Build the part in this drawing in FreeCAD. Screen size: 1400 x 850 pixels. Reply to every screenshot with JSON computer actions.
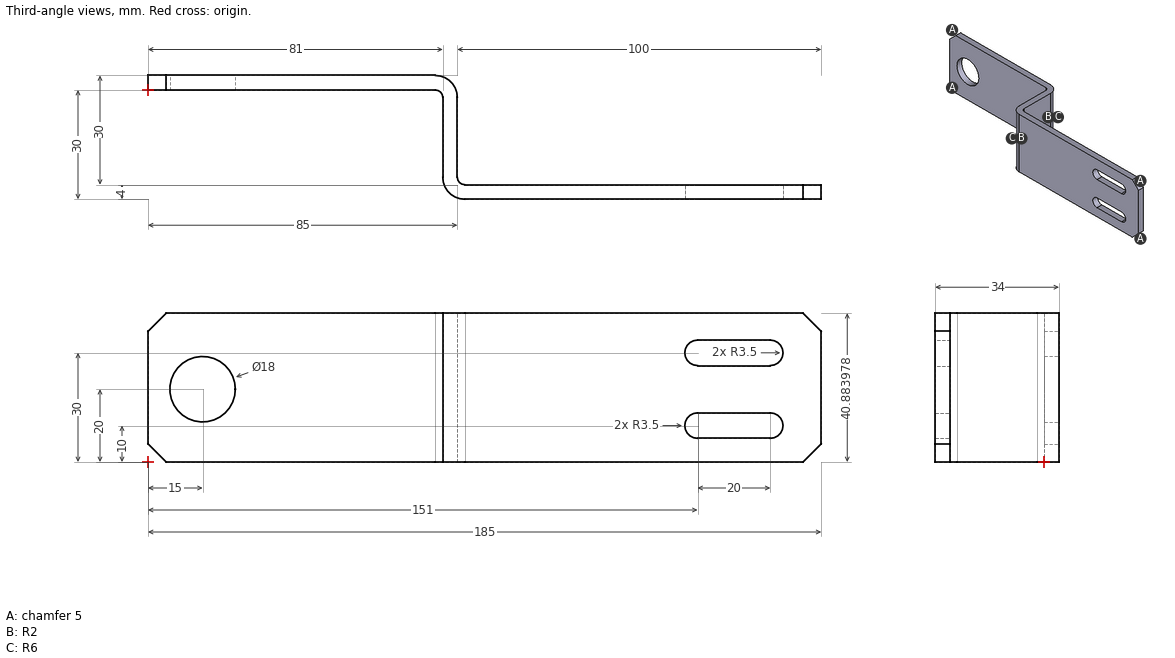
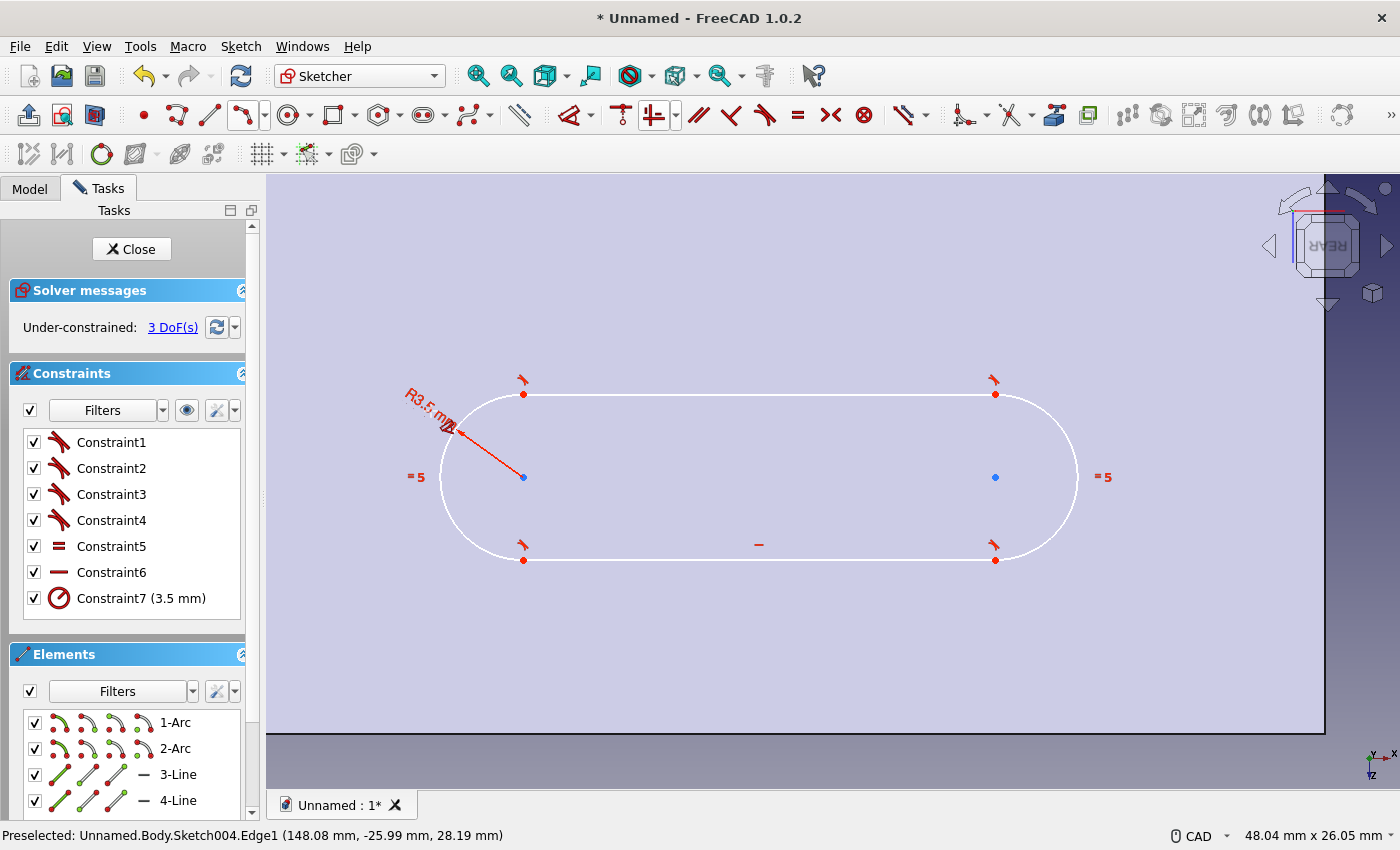
{"action": "left_click", "coordinate": [665, 395]}
{"action": "left_click", "coordinate": [759, 361]}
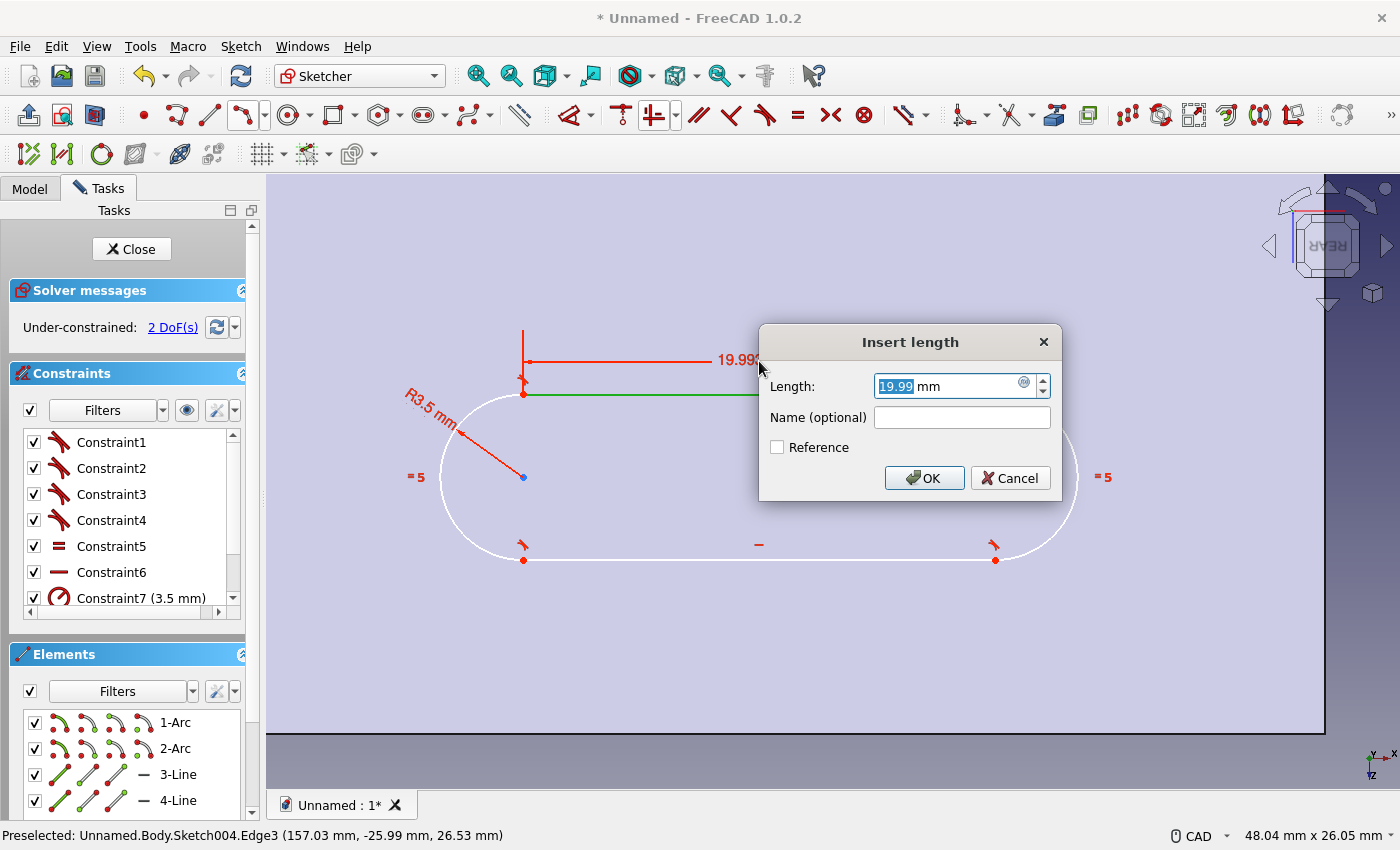
{"action": "type", "text": "20"}
{"action": "key", "text": "Return"}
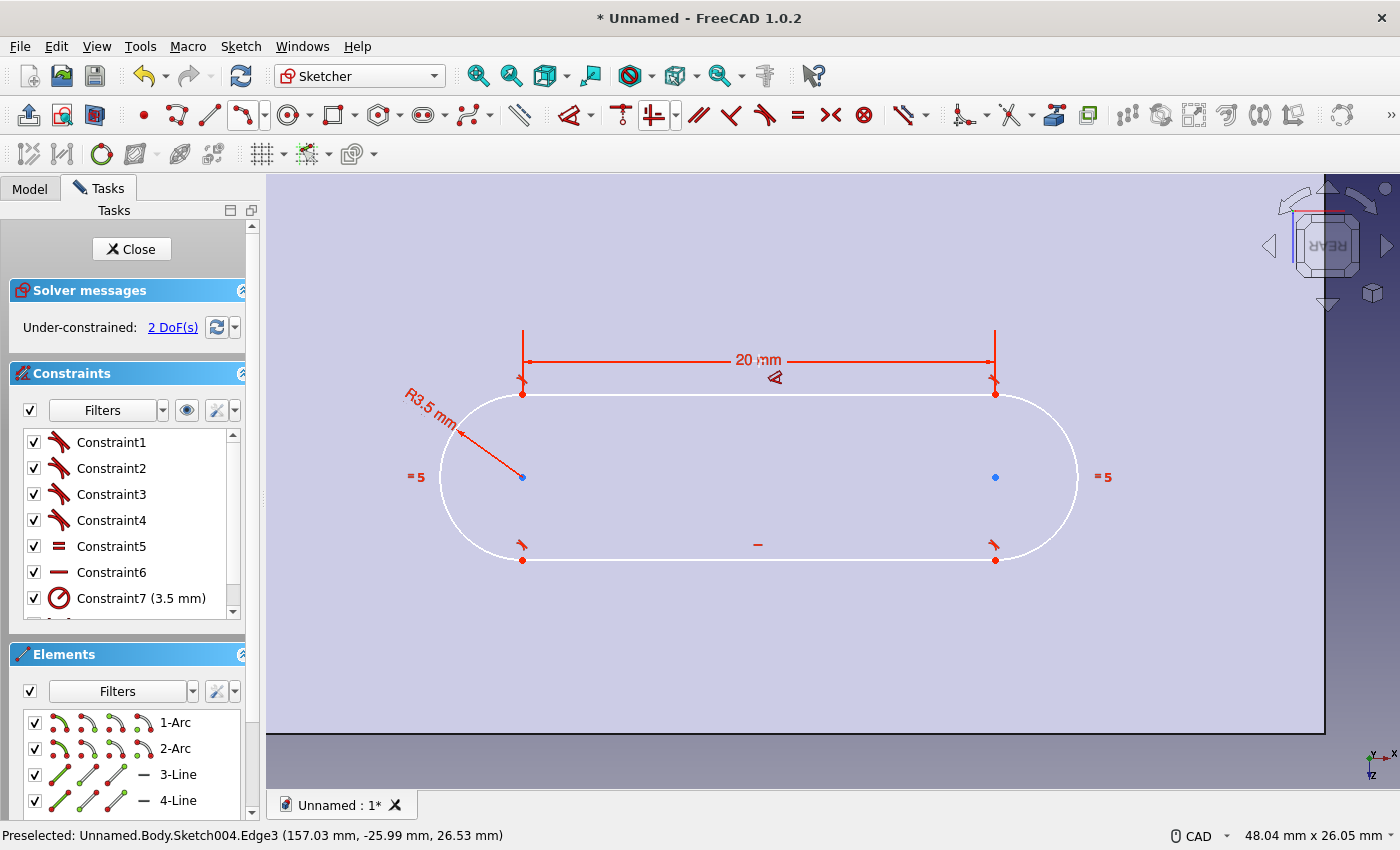
{"action": "left_click", "coordinate": [523, 477]}
{"action": "left_click", "coordinate": [557, 340]}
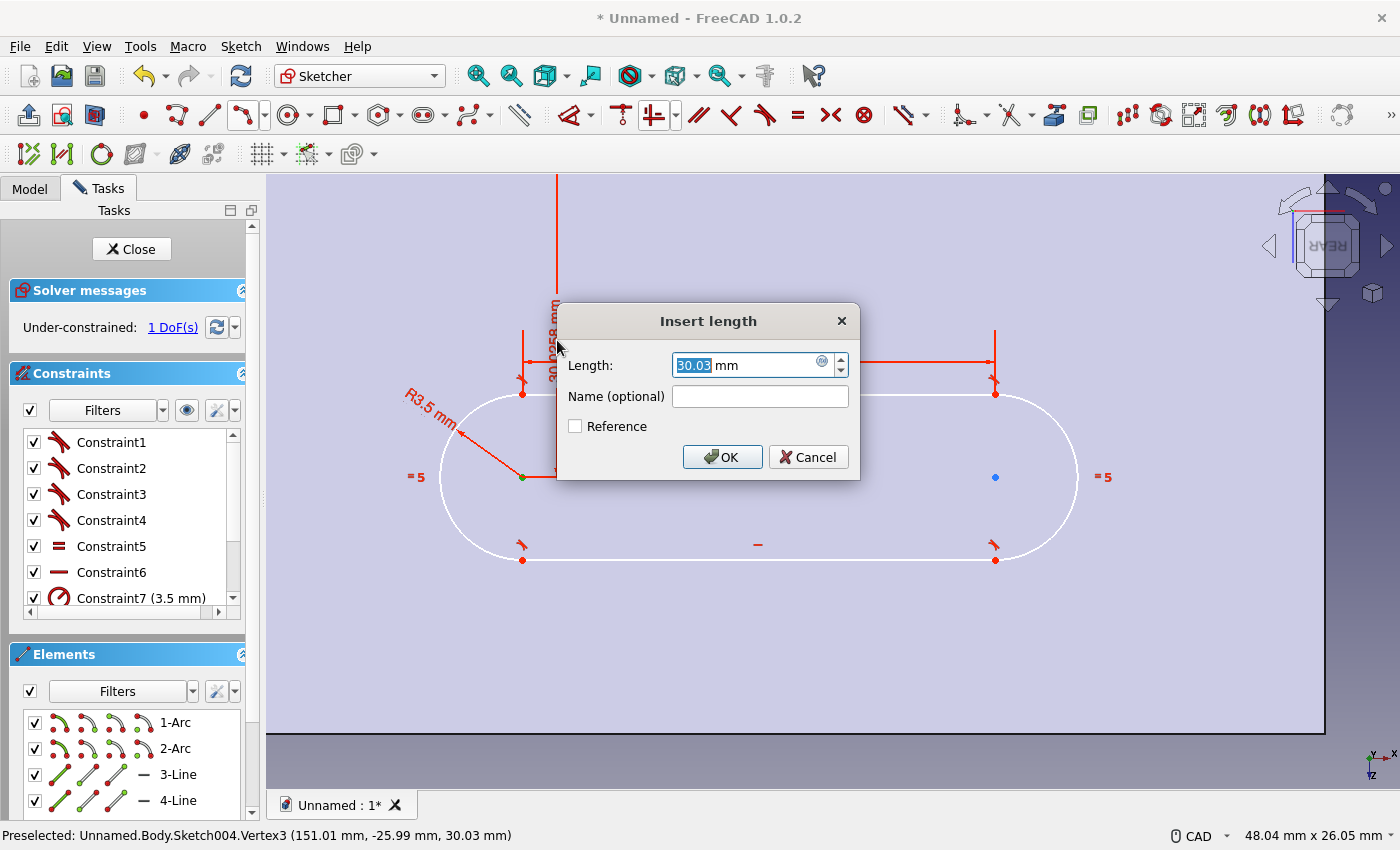
{"action": "type", "text": "30"}
{"action": "key", "text": "Return"}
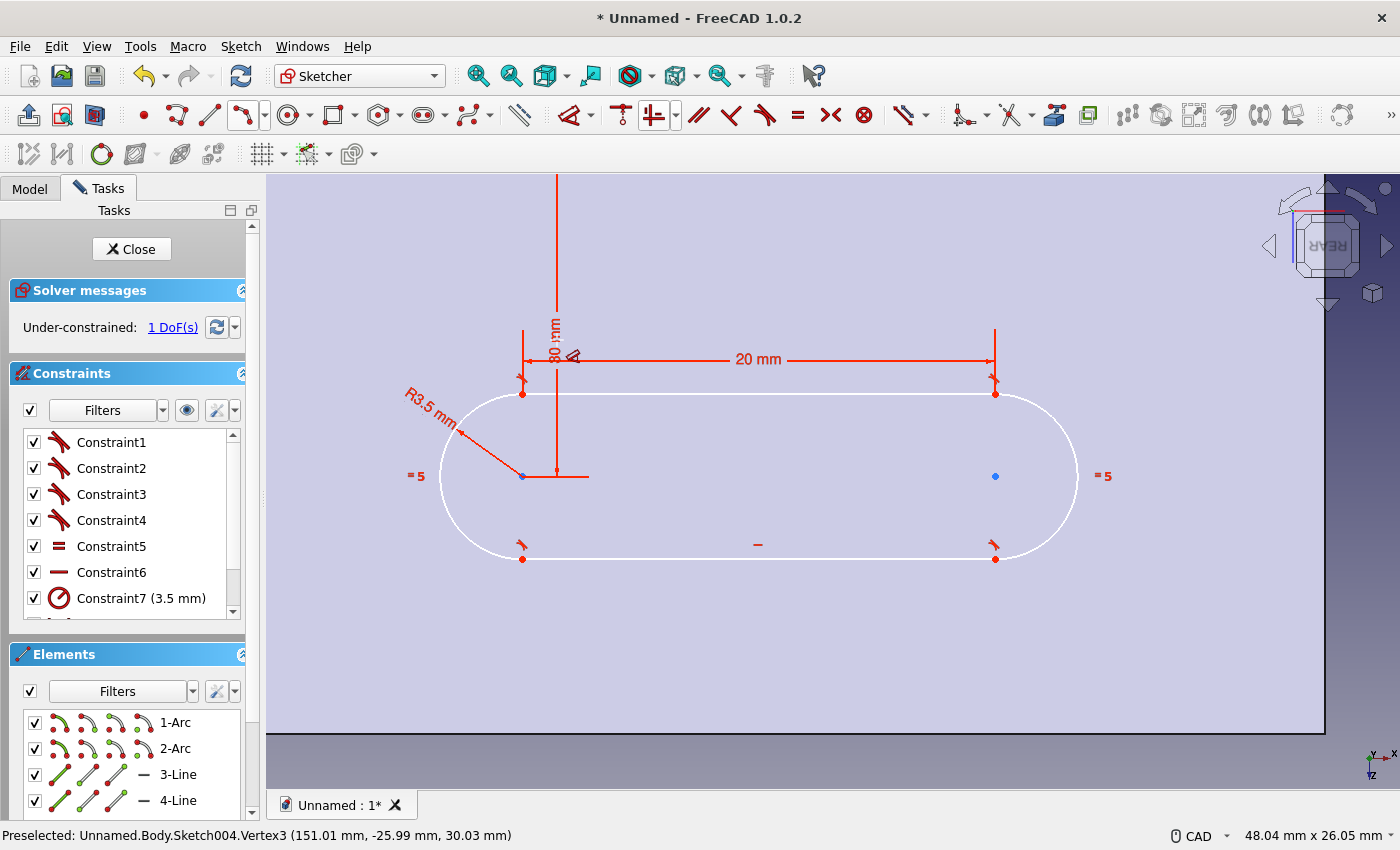
{"action": "left_click", "coordinate": [523, 394]}
{"action": "left_click", "coordinate": [356, 428]}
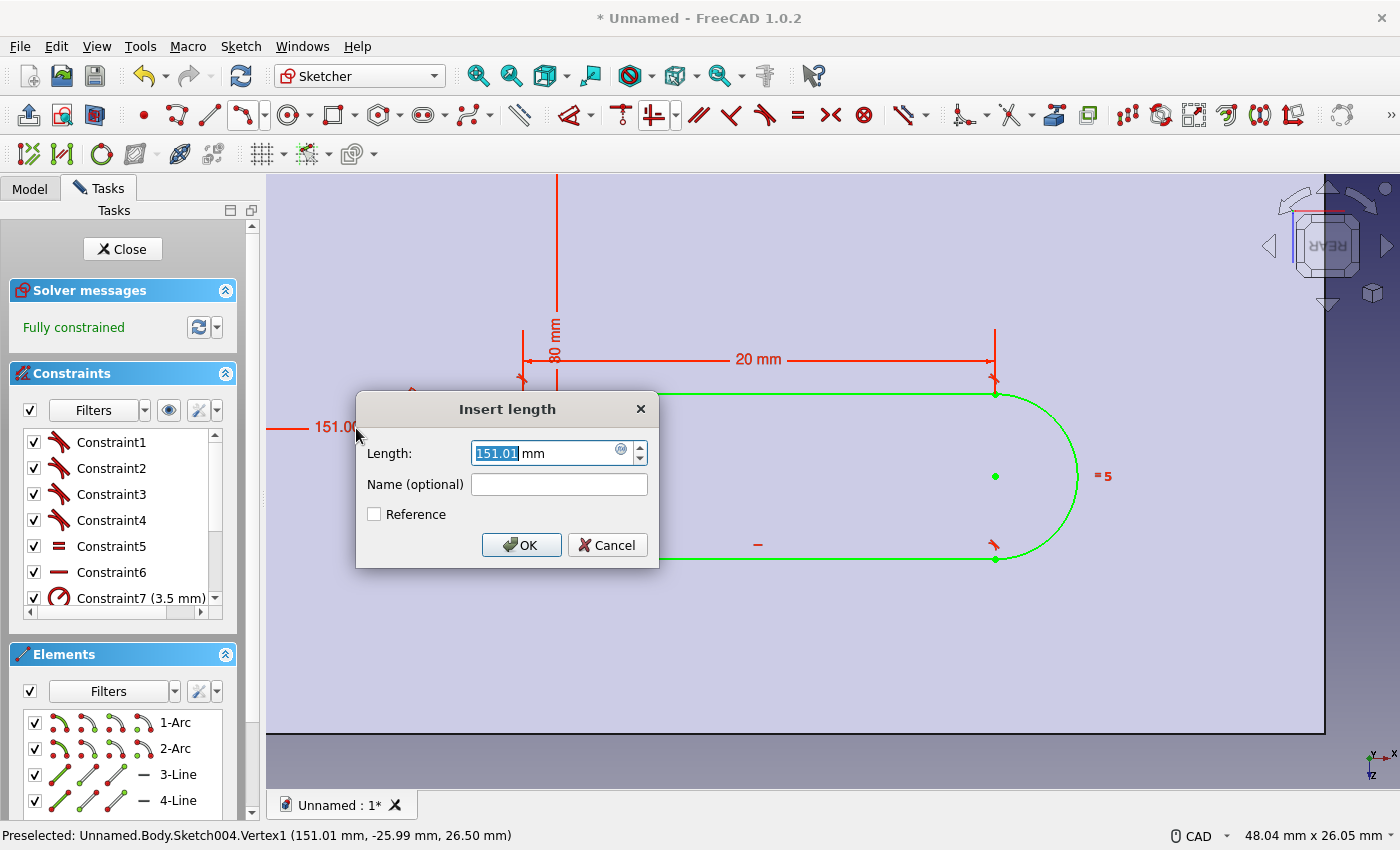
{"action": "type", "text": "151"}
{"action": "key", "text": "Return"}
{"action": "key", "text": "Escape"}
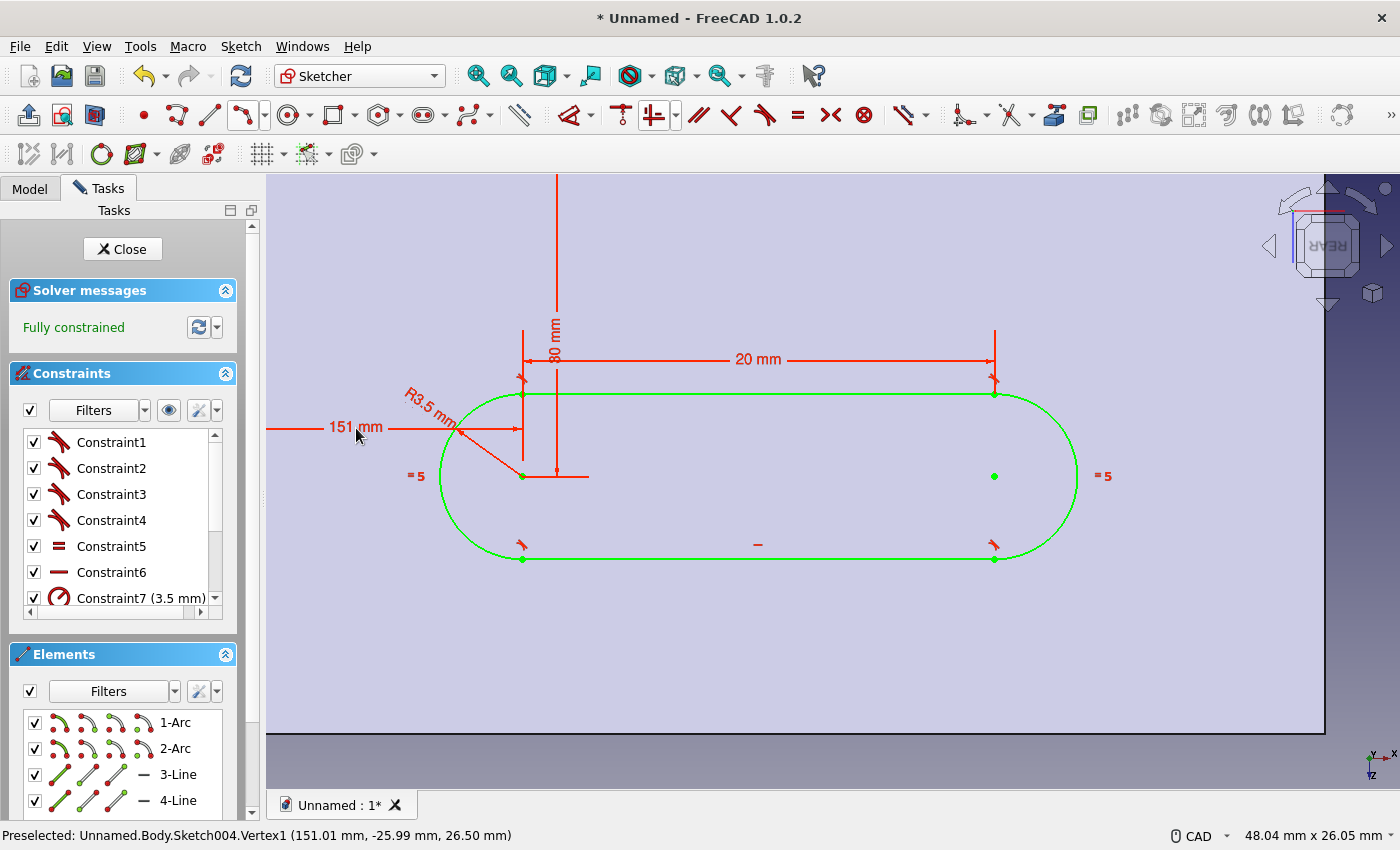
{"action": "left_click", "coordinate": [123, 249]}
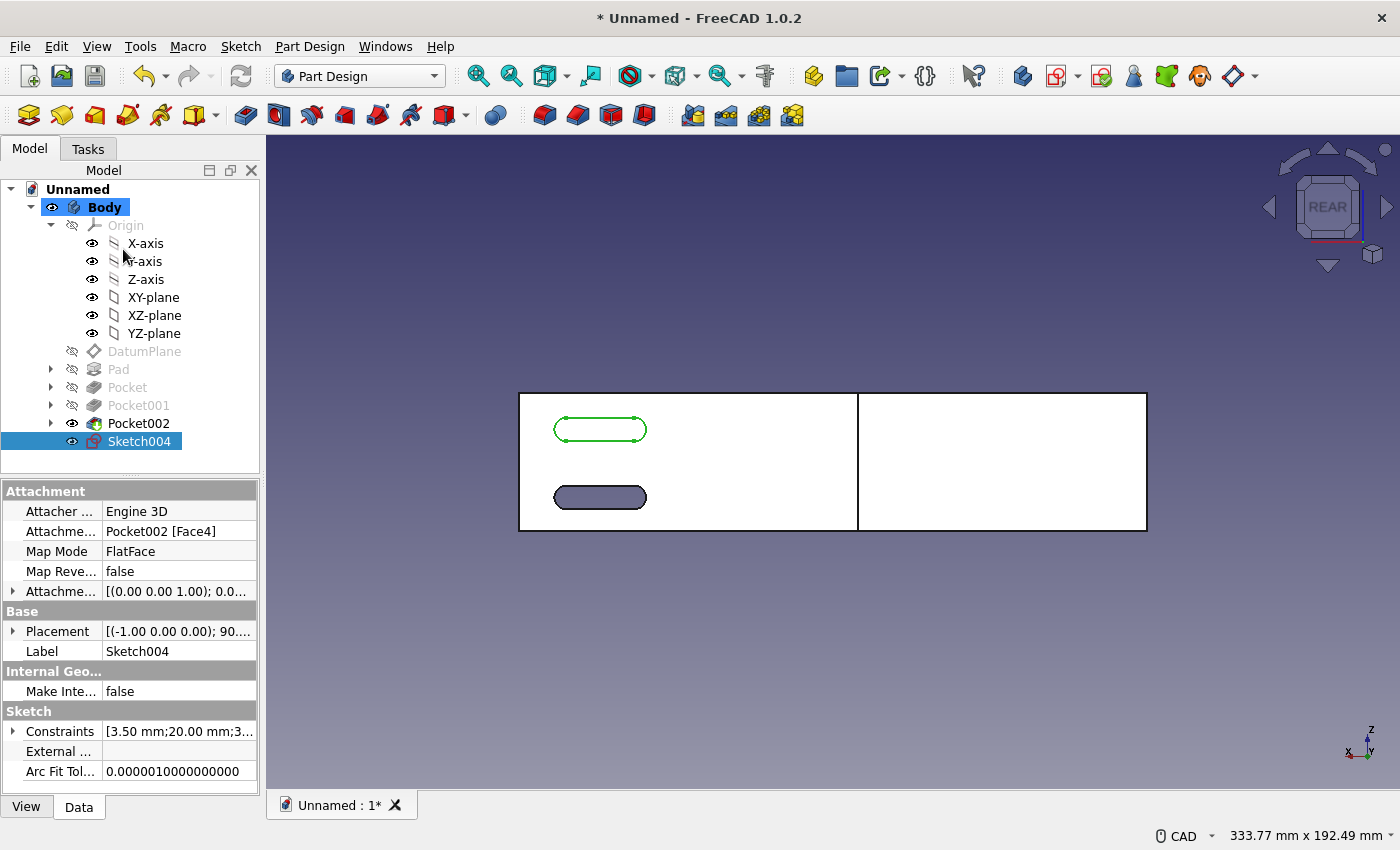
{"action": "left_click", "coordinate": [246, 116]}